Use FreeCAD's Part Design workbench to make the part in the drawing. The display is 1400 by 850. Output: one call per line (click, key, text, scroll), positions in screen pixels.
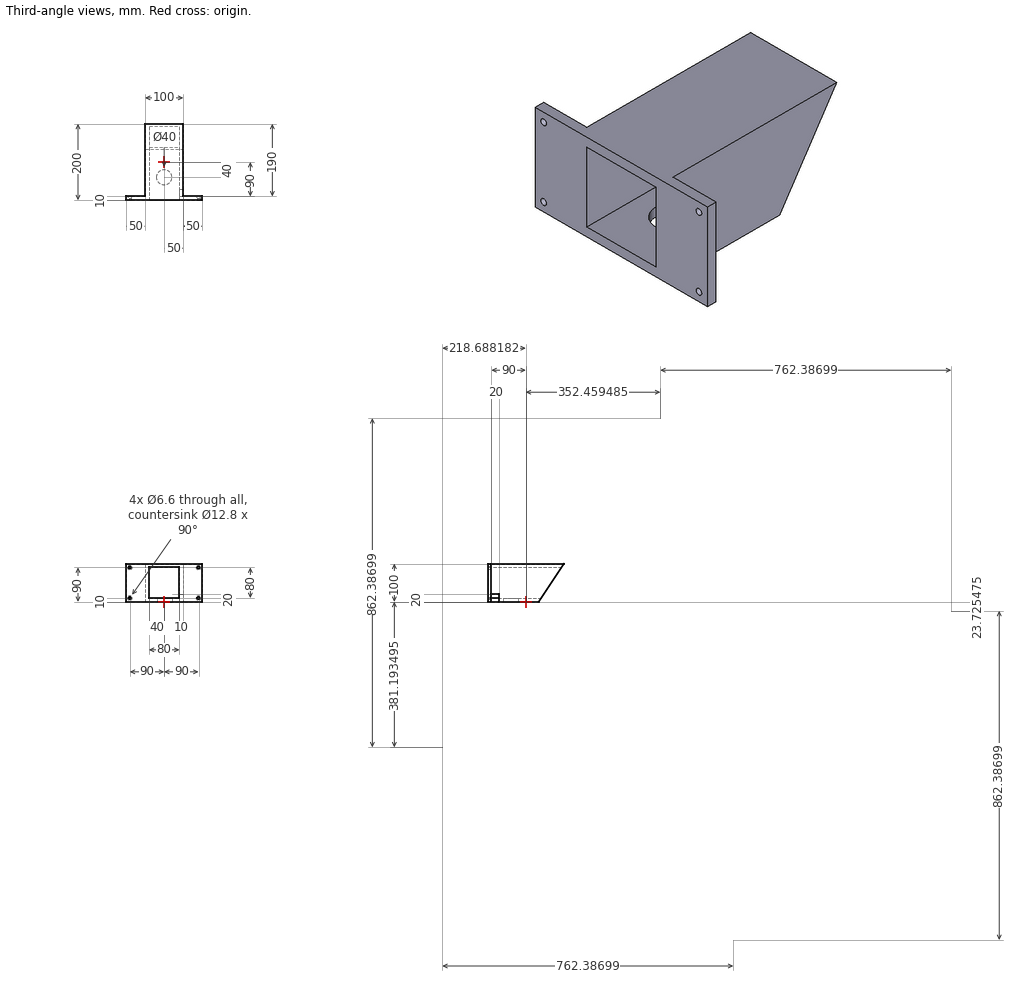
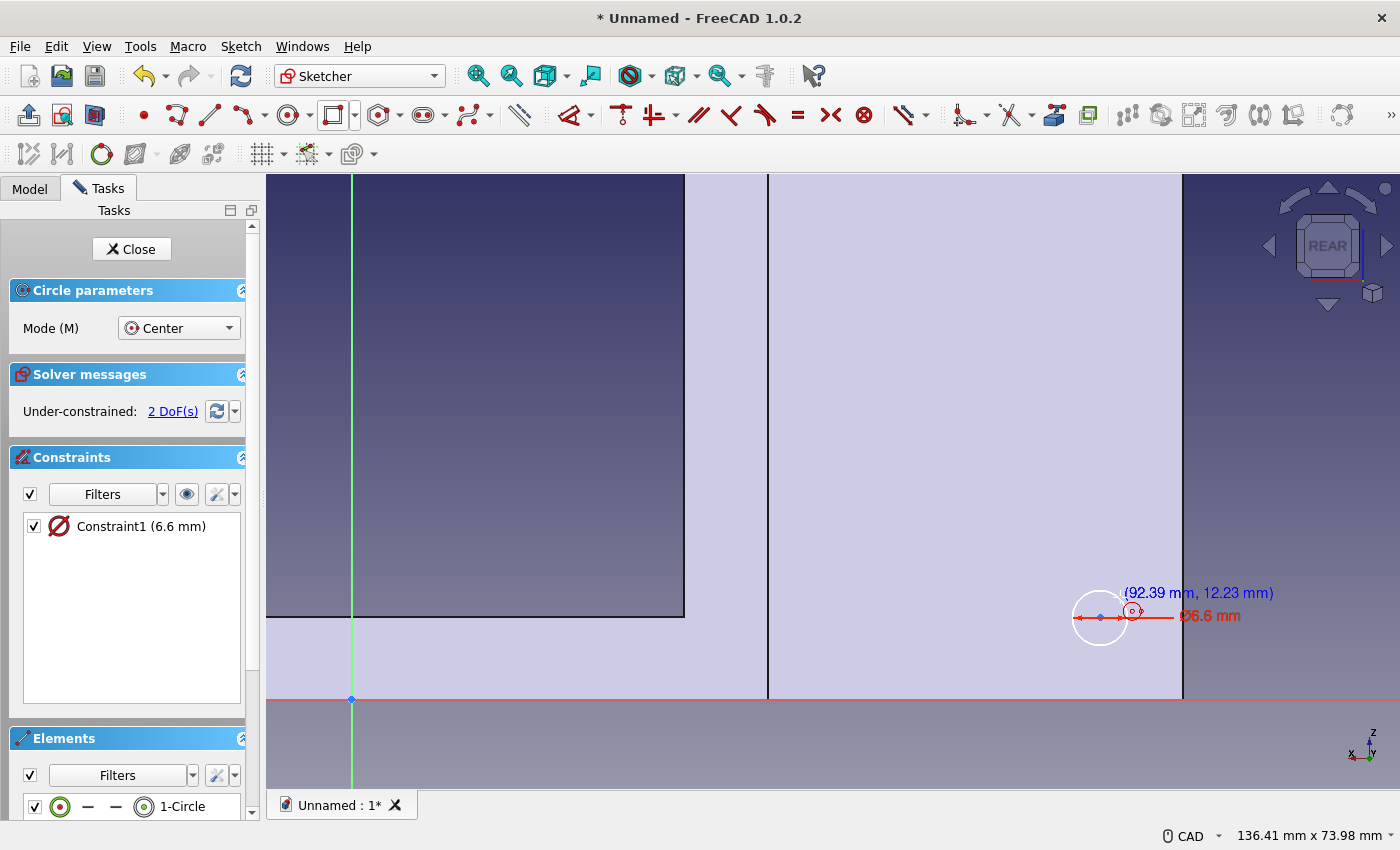
scroll(1101, 620, down, 4)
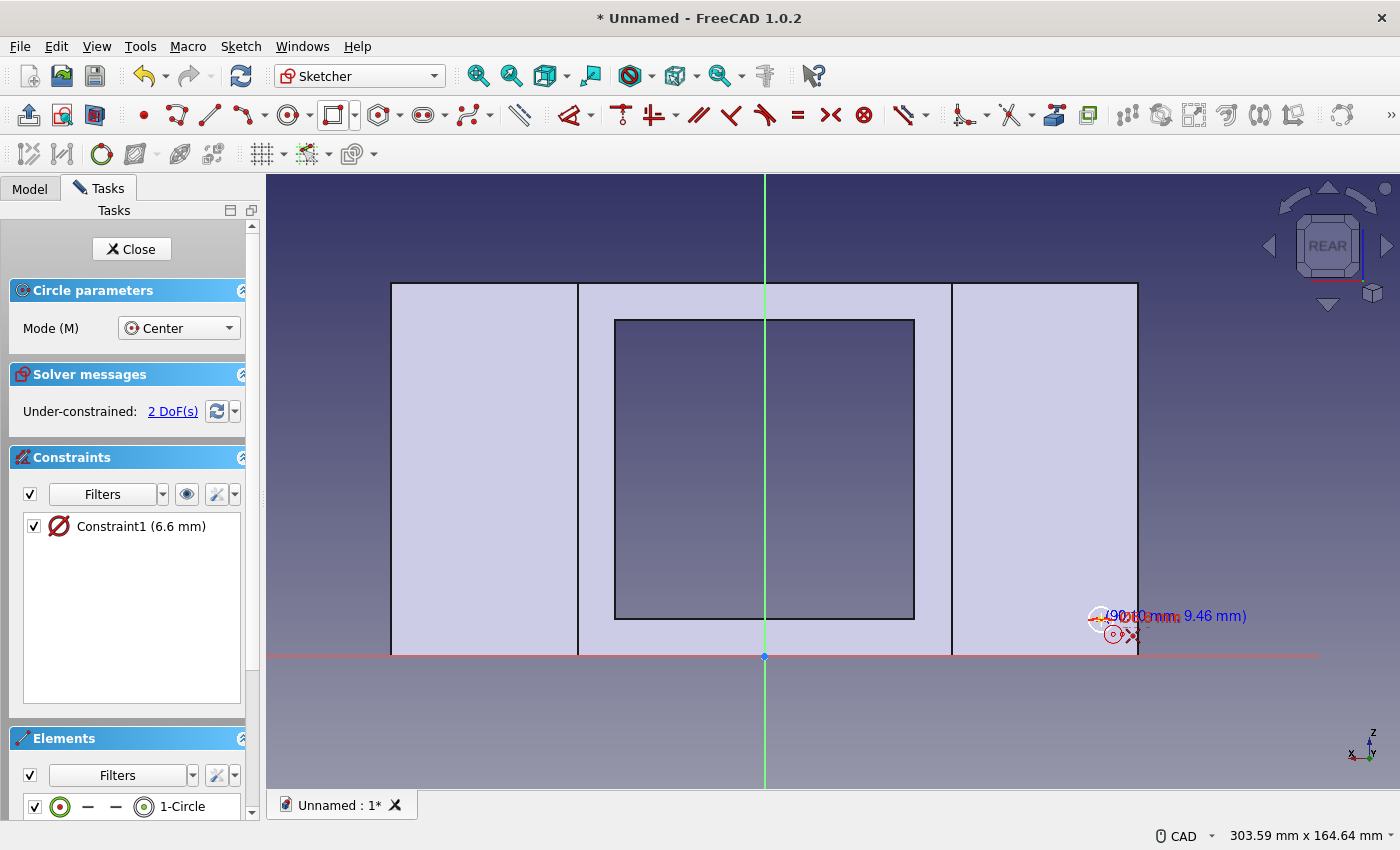
scroll(1101, 320, up, 4)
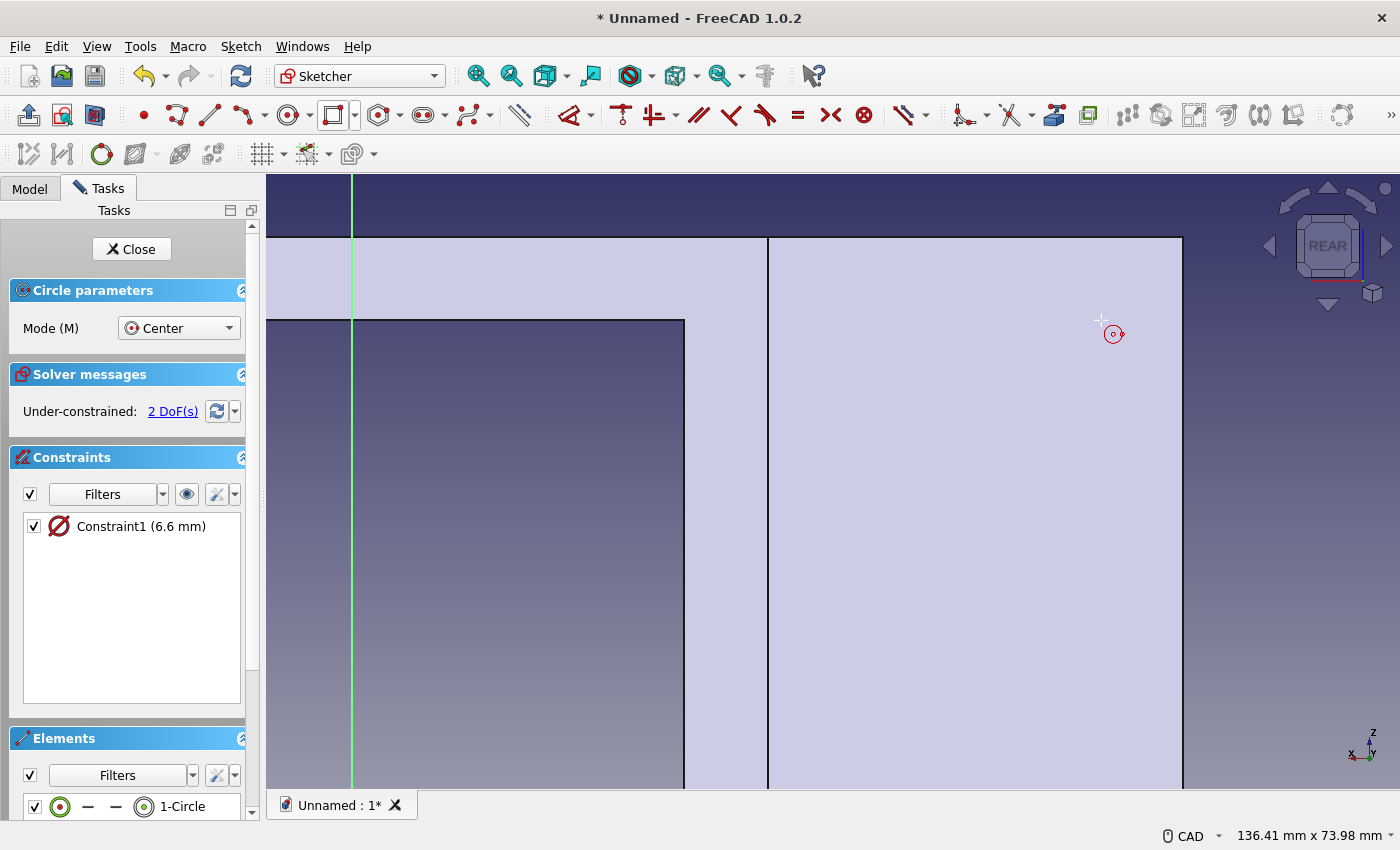
click(1100, 320)
move(1120, 300)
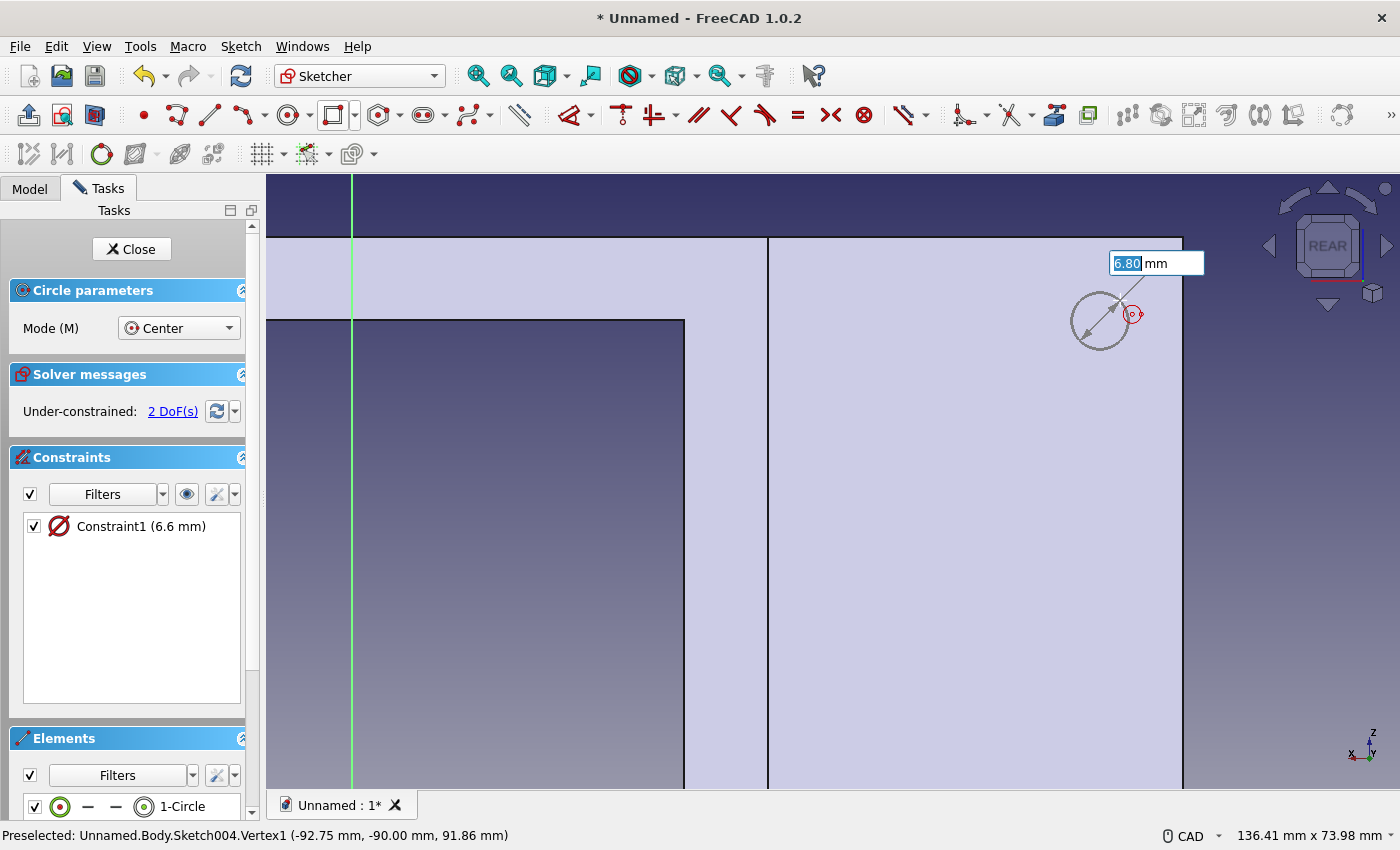
text(6.6)
key(Return)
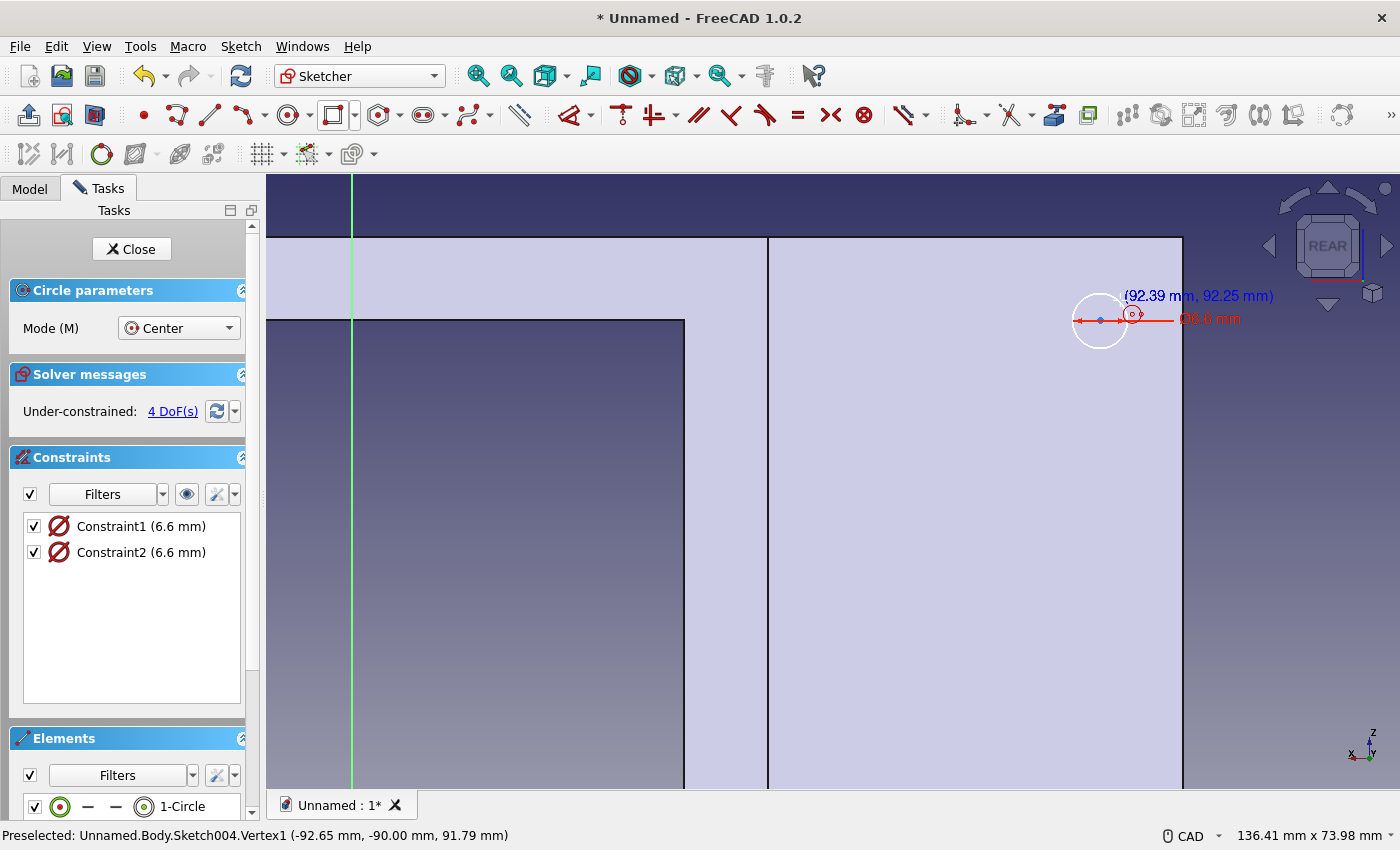
scroll(1101, 319, down, 4)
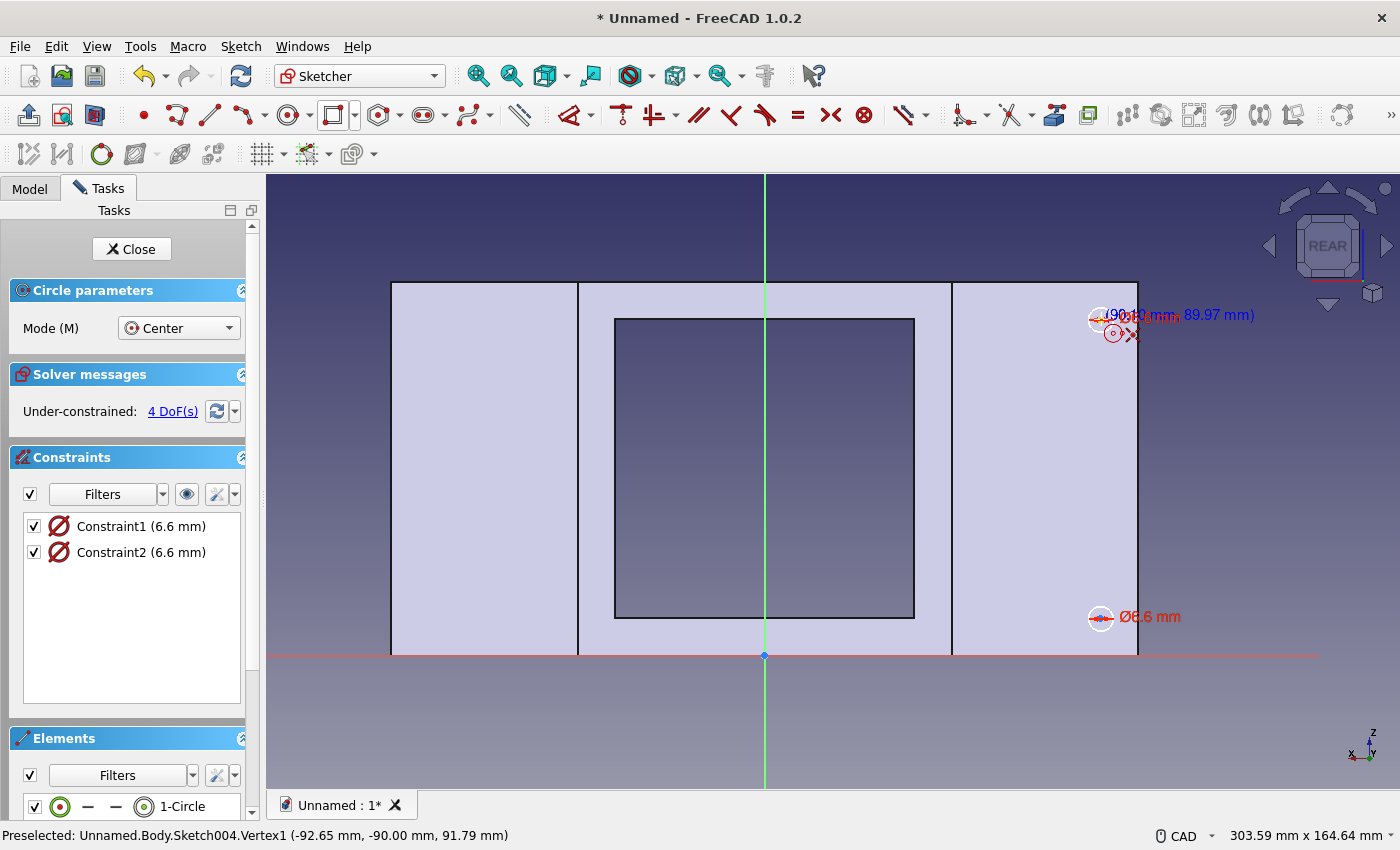
scroll(429, 618, up, 4)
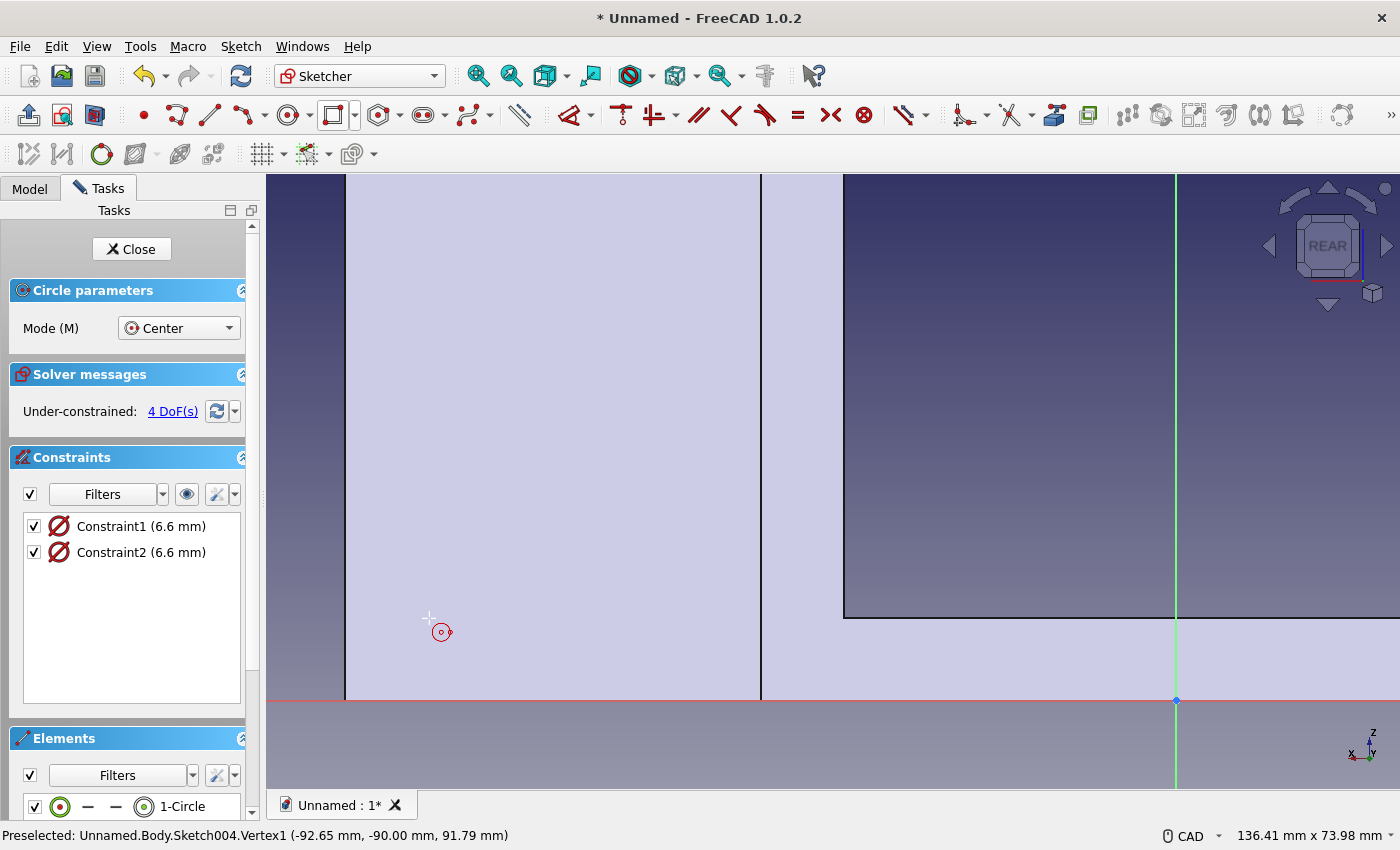
click(428, 618)
move(447, 598)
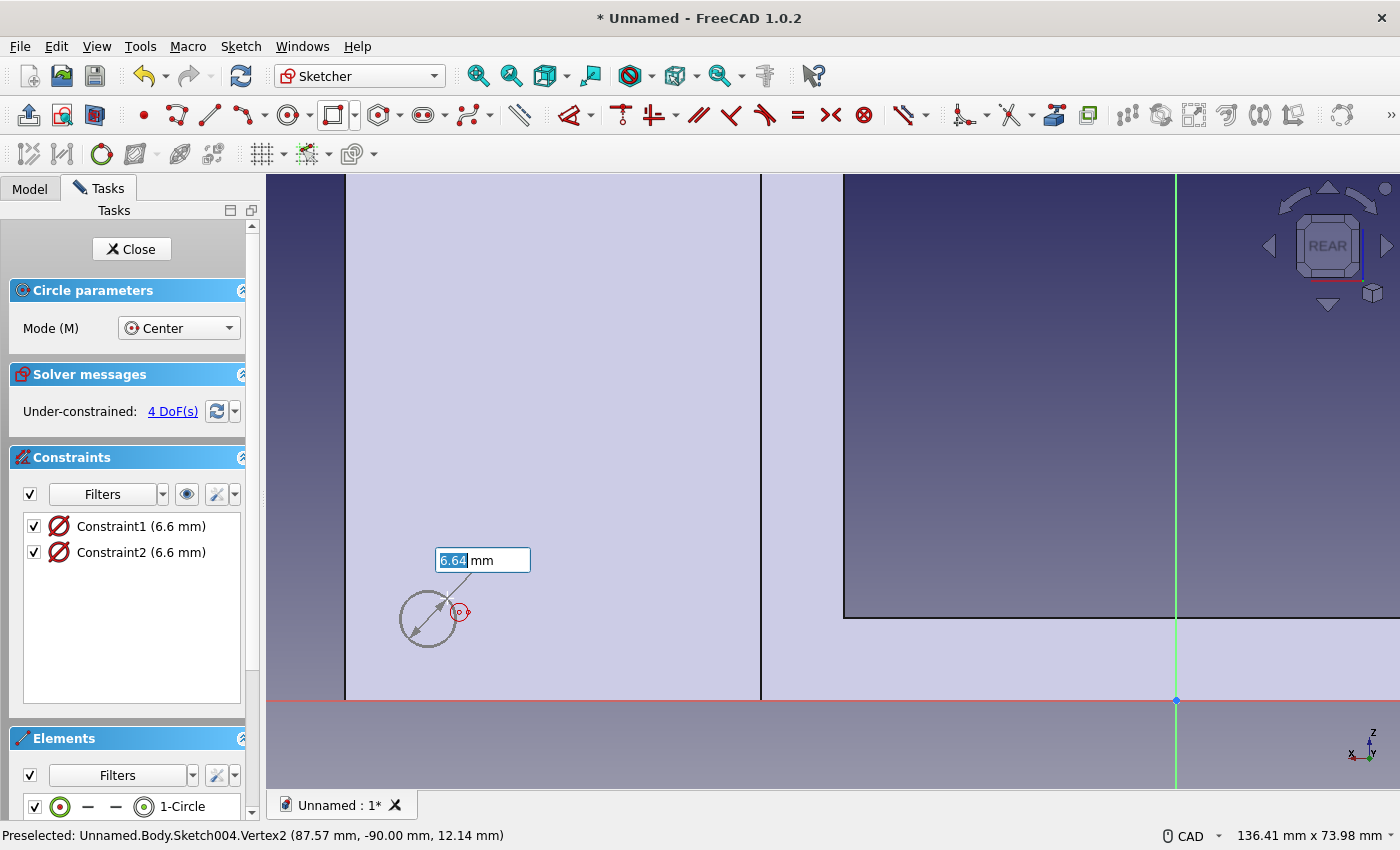
text(6.6)
key(Return)